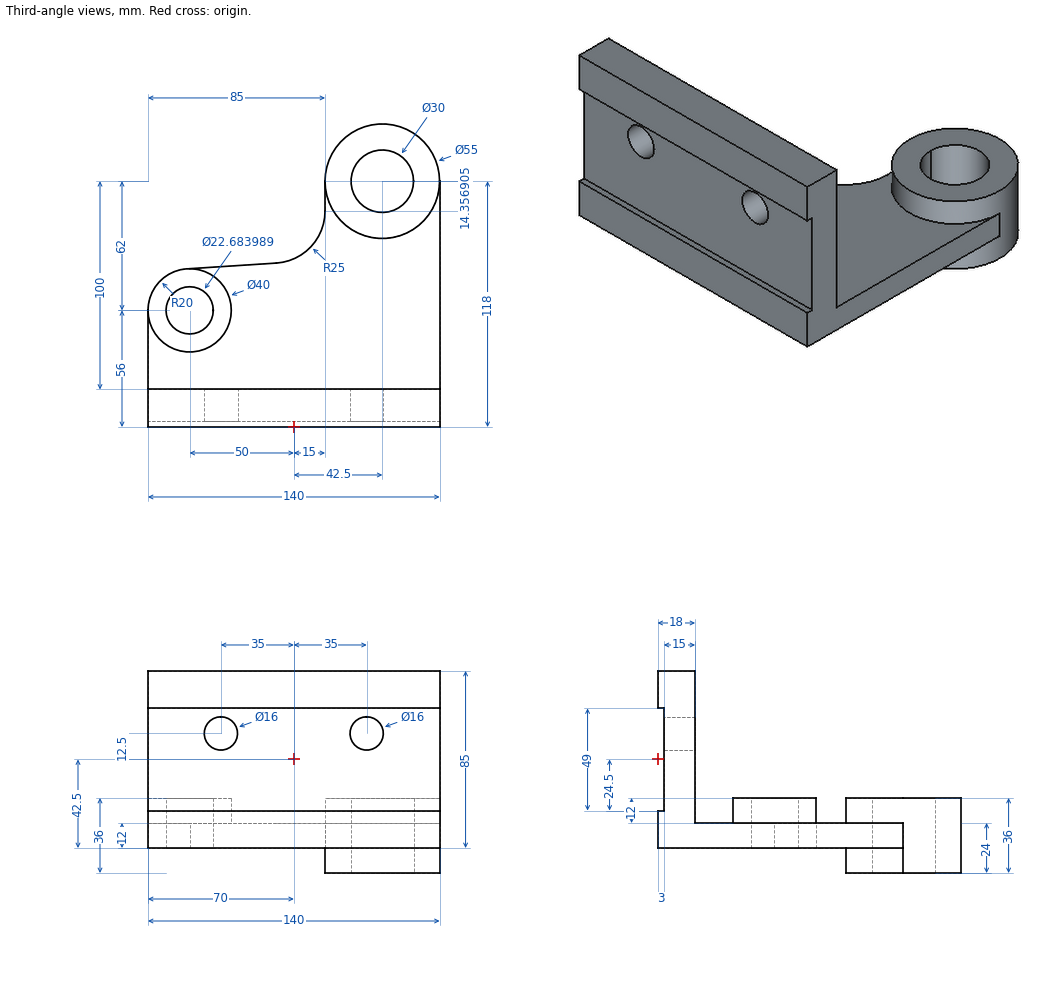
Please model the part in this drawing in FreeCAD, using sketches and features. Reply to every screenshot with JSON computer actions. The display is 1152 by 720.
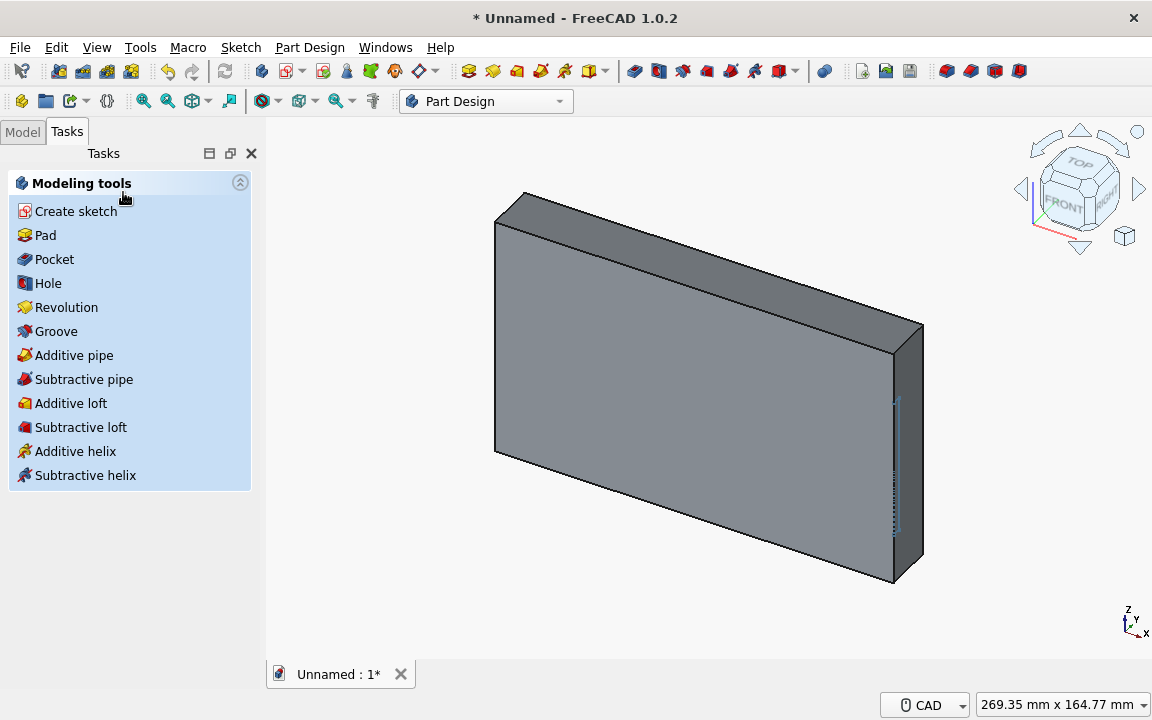
{"action": "left_click", "coordinate": [636, 72]}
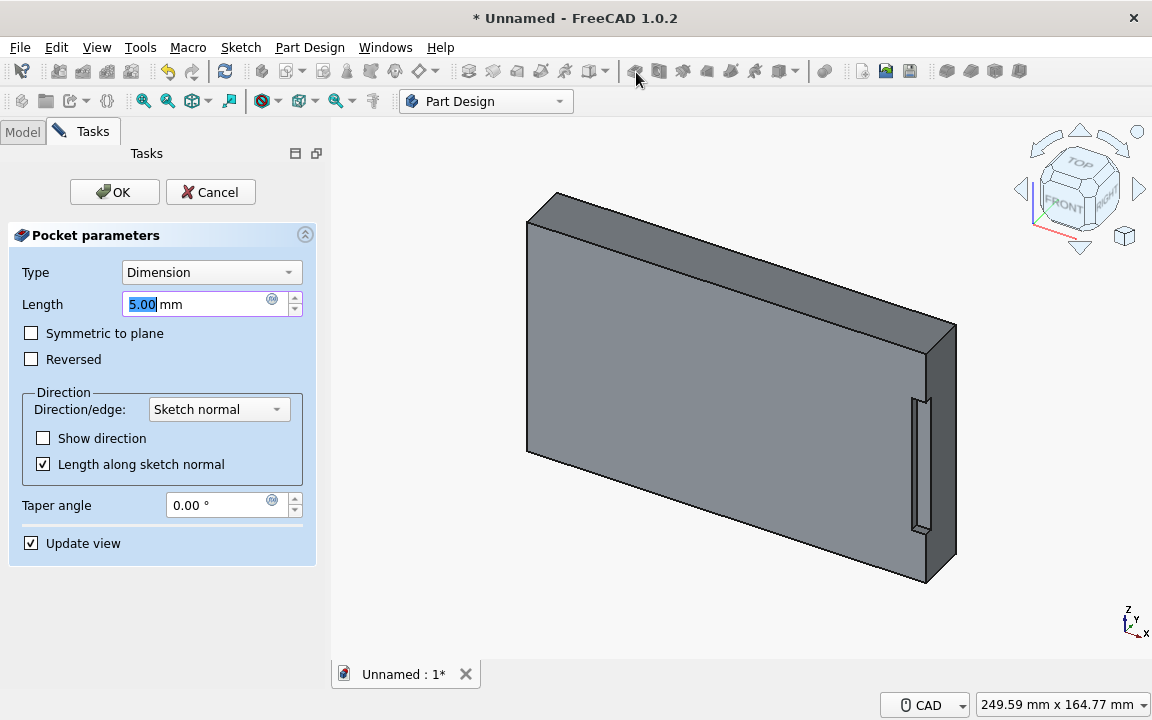
{"action": "type", "text": "140"}
{"action": "key", "text": "Tab"}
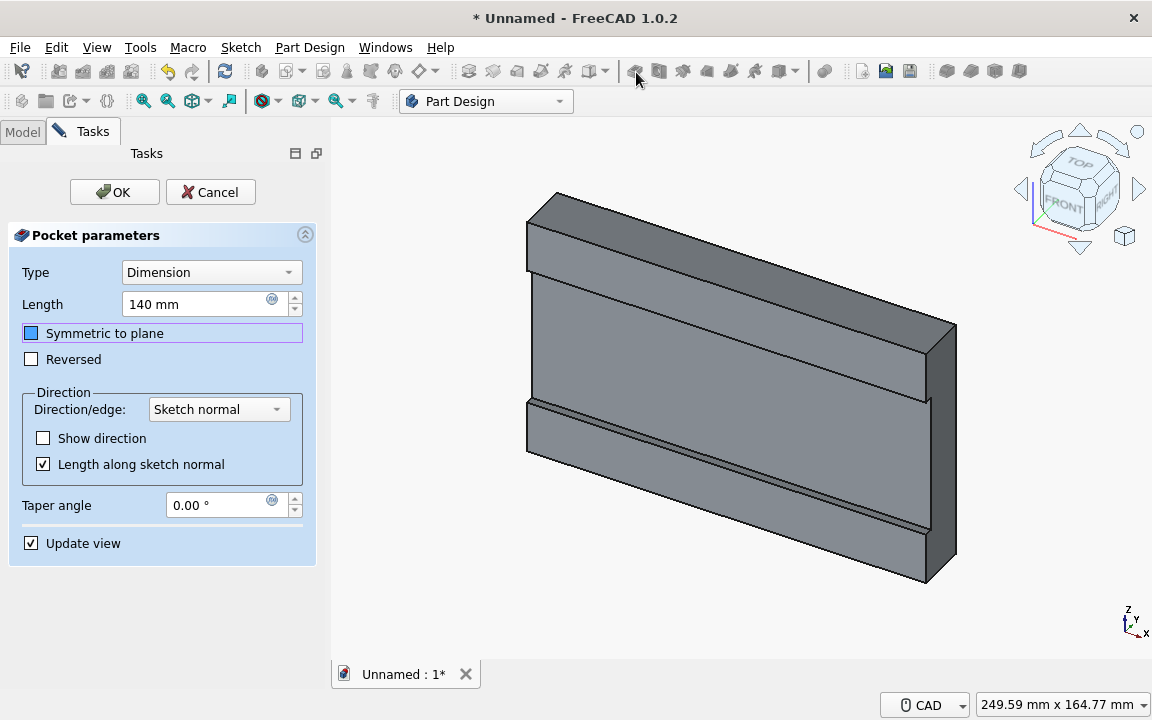
{"action": "left_click", "coordinate": [115, 192]}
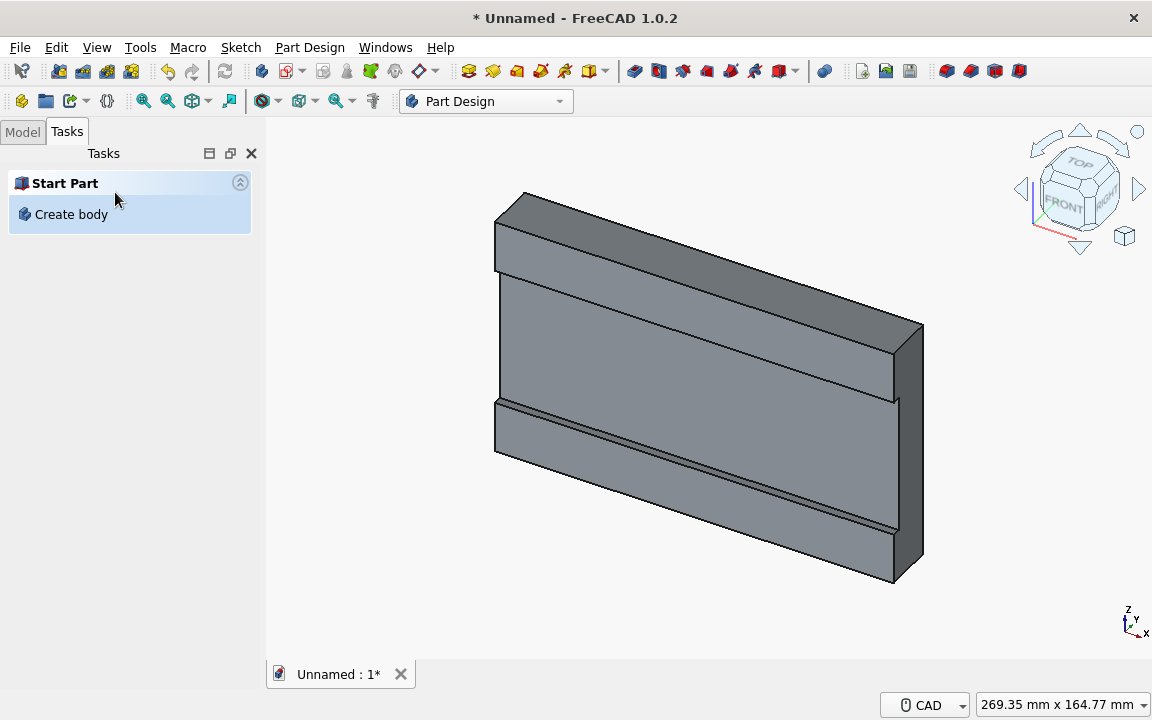
{"action": "key", "text": "4"}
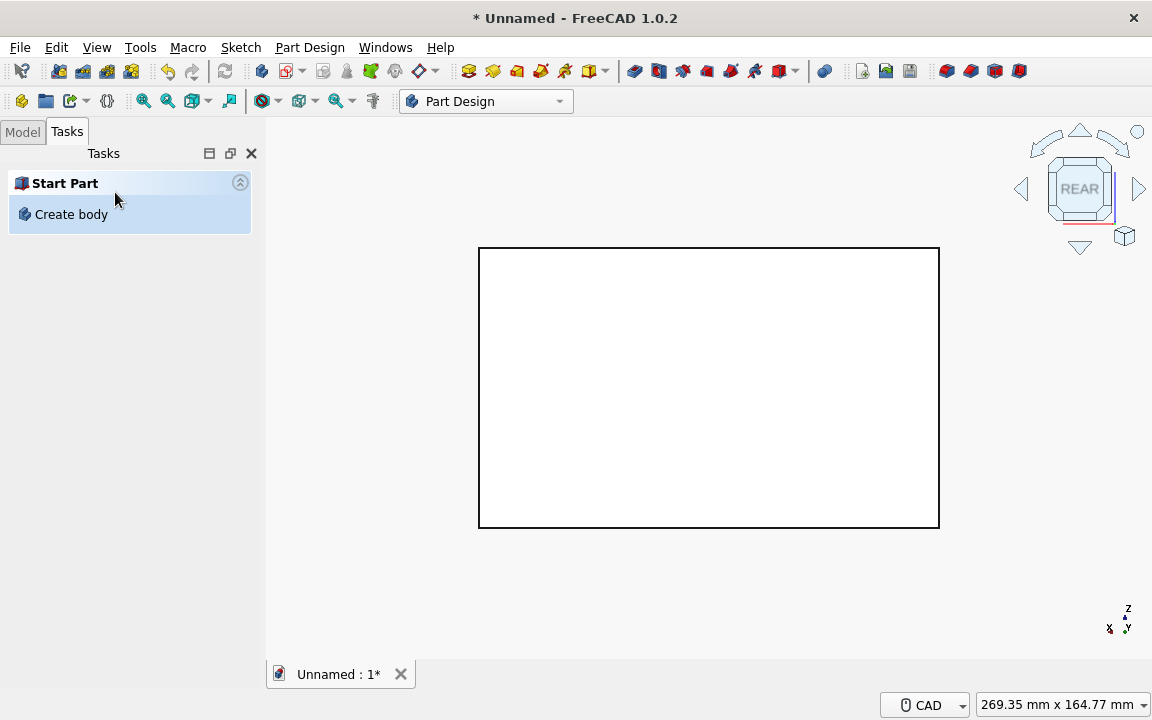
{"action": "left_click", "coordinate": [643, 387]}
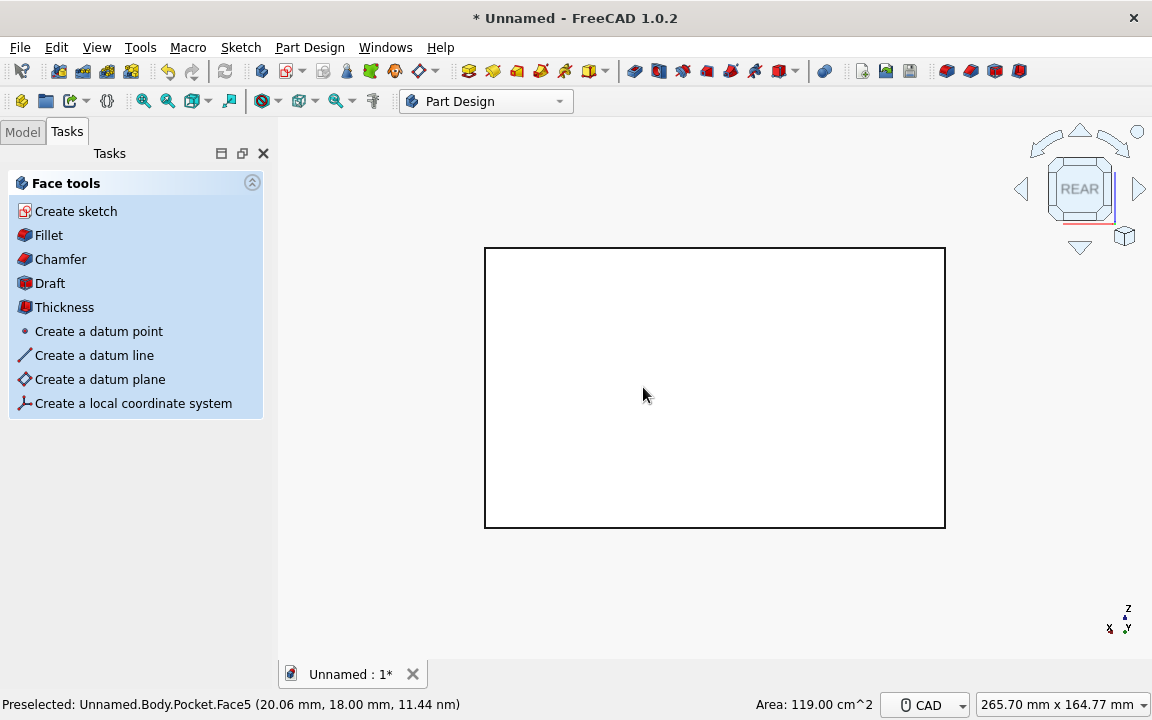
{"action": "left_click", "coordinate": [286, 72]}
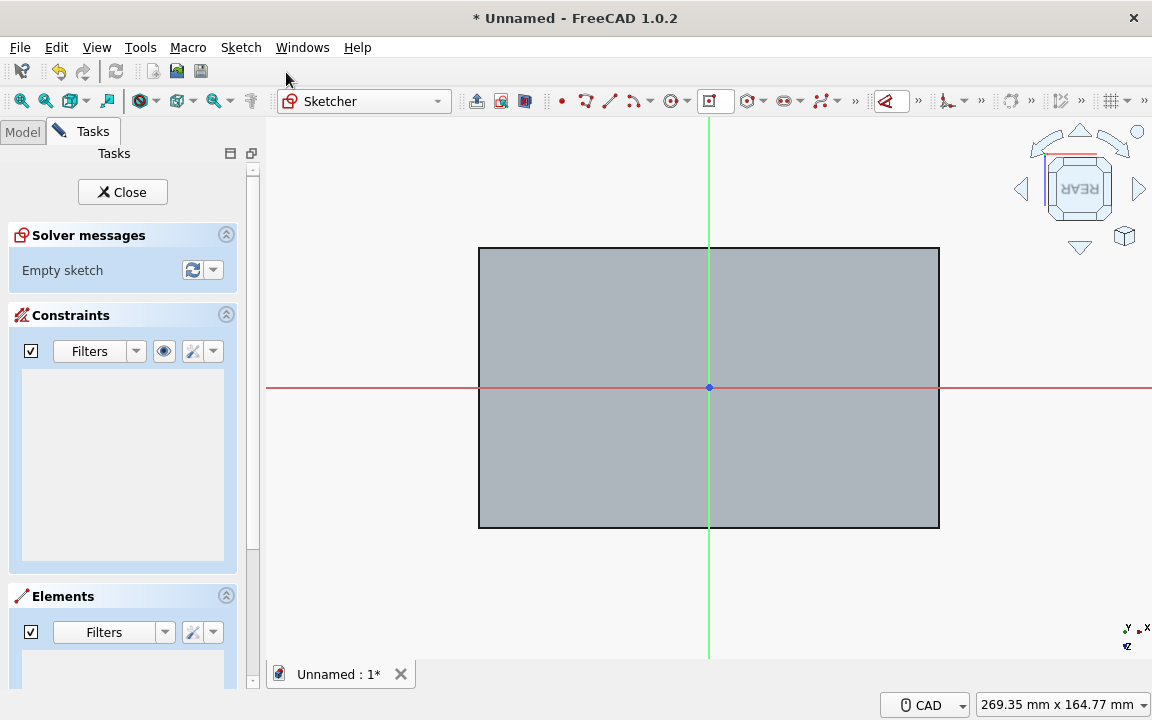
{"action": "key", "text": "g r"}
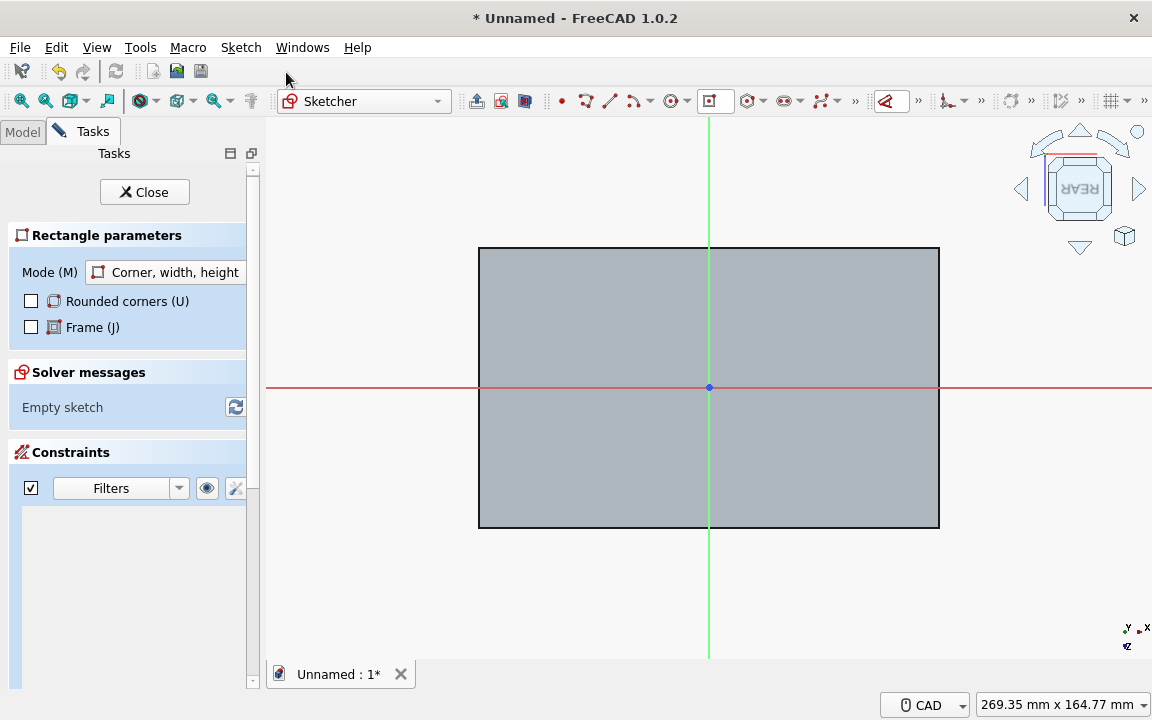
{"action": "left_click", "coordinate": [479, 248]}
{"action": "left_click", "coordinate": [939, 288]}
{"action": "key", "text": "Escape"}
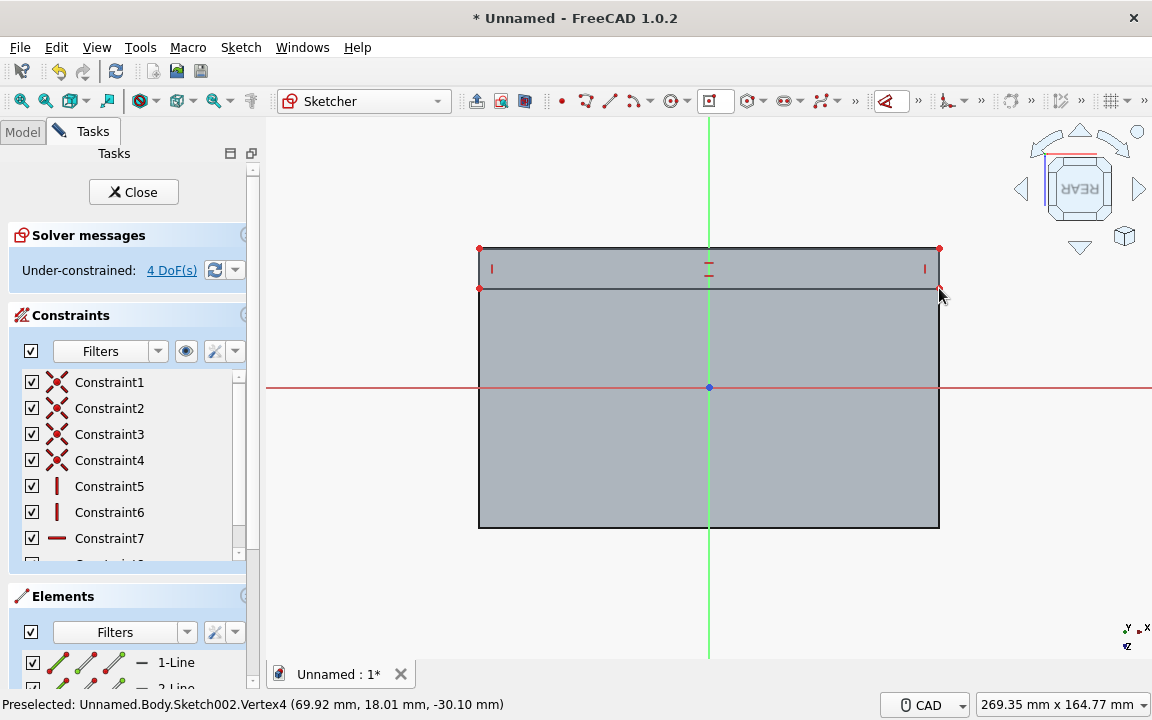
{"action": "left_click", "coordinate": [479, 261]}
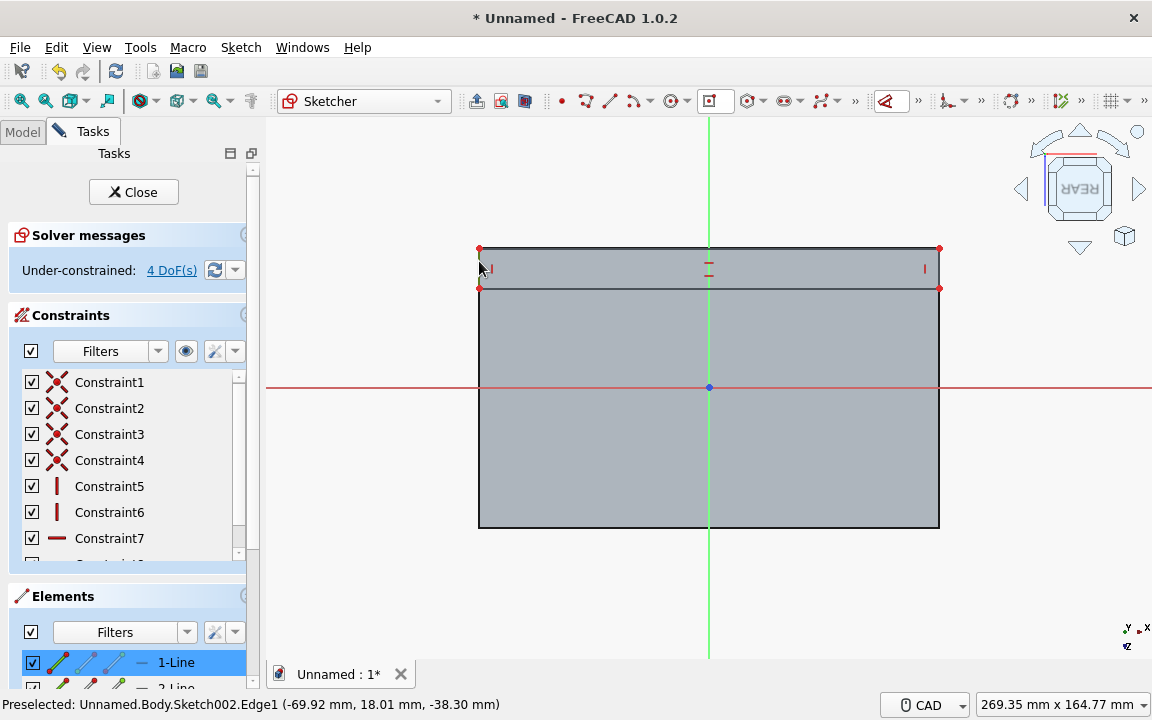
{"action": "key", "text": "i"}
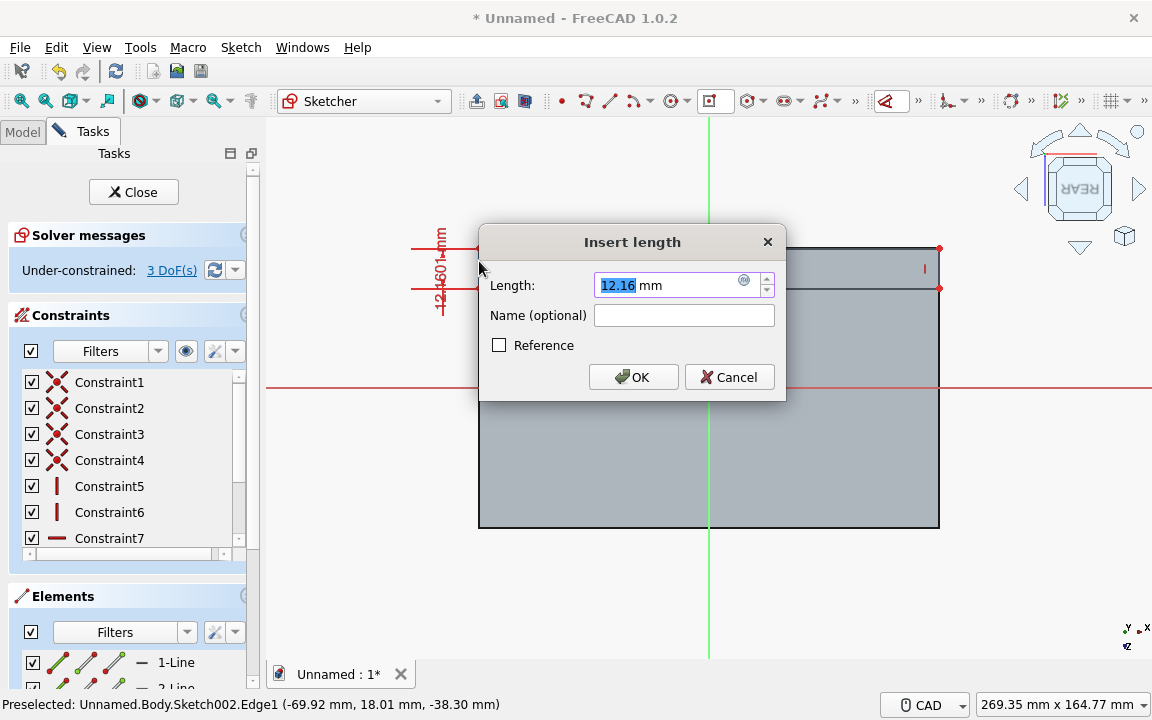
{"action": "type", "text": "12"}
{"action": "key", "text": "Return"}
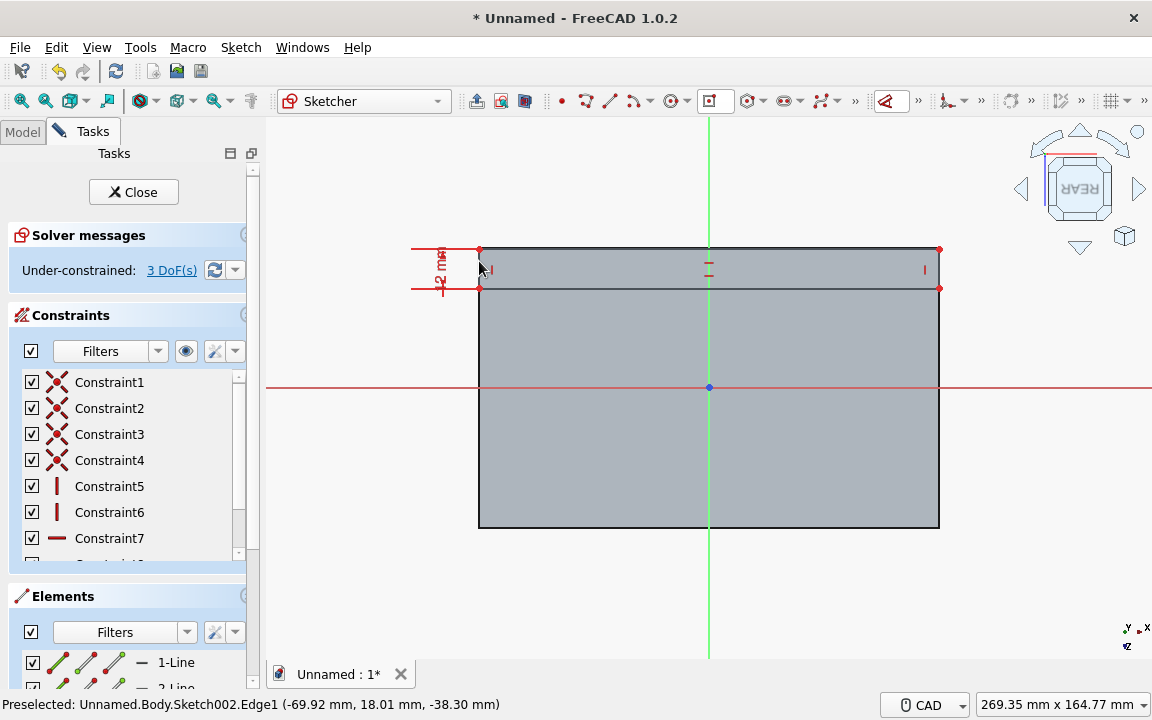
{"action": "left_click", "coordinate": [617, 289]}